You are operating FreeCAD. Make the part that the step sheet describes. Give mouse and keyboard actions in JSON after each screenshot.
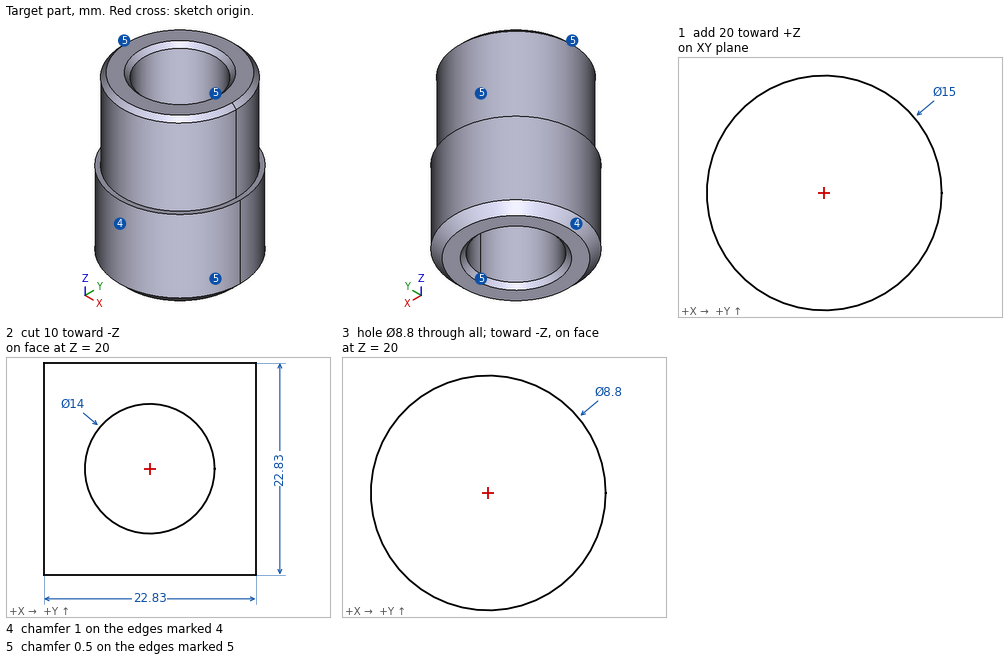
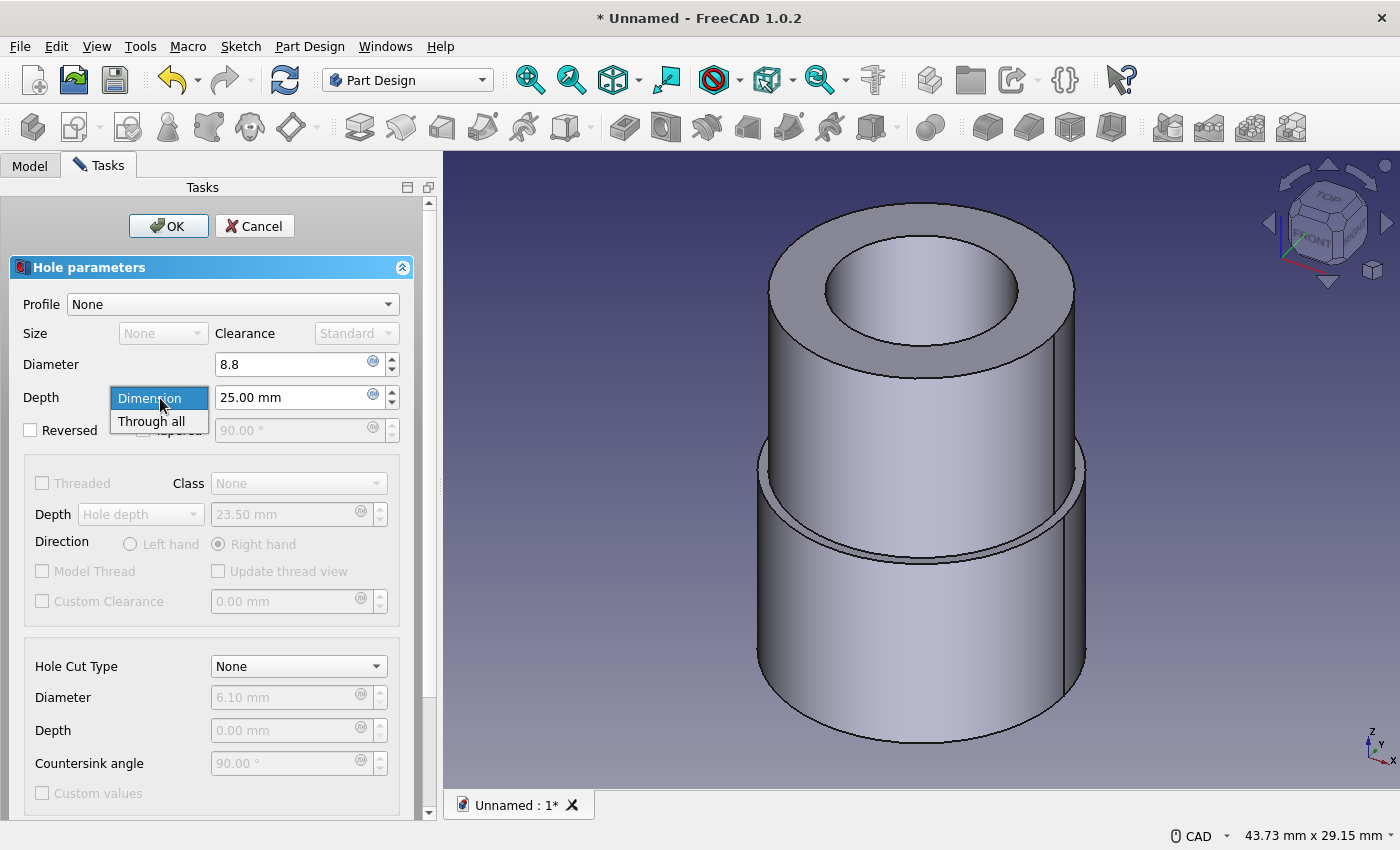
{"action": "left_click", "coordinate": [158, 422]}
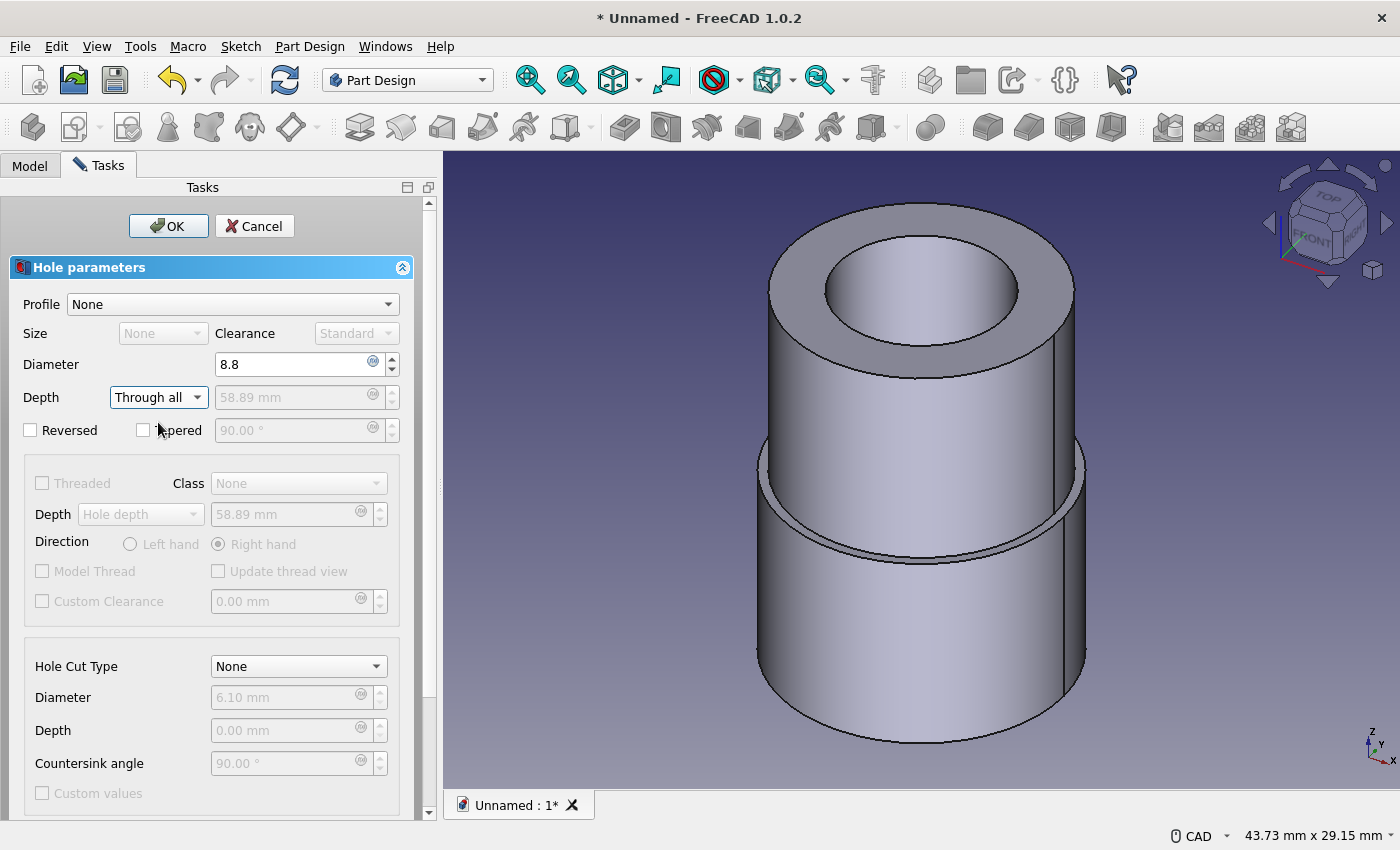
{"action": "left_click", "coordinate": [169, 226]}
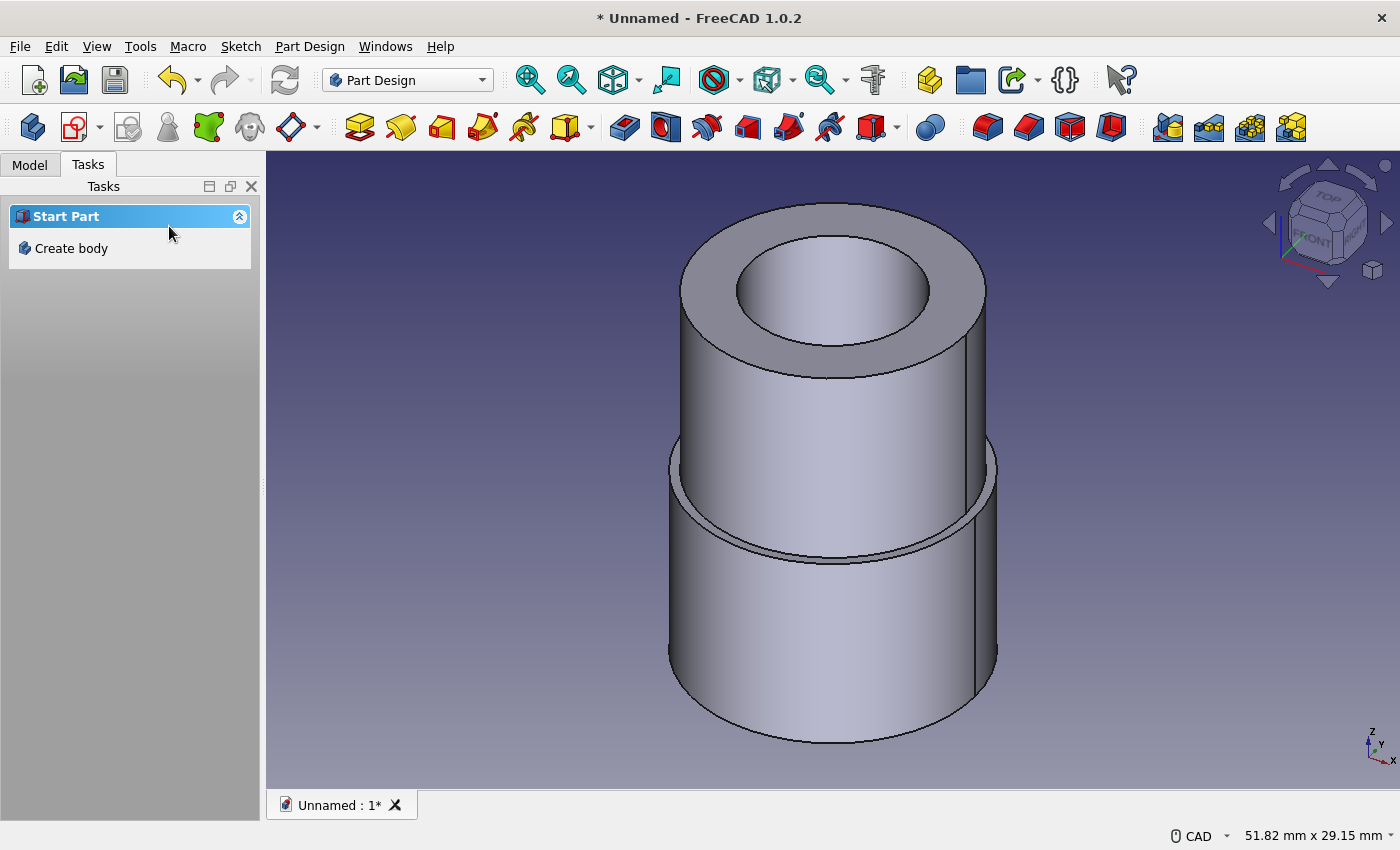
{"action": "key", "text": "0"}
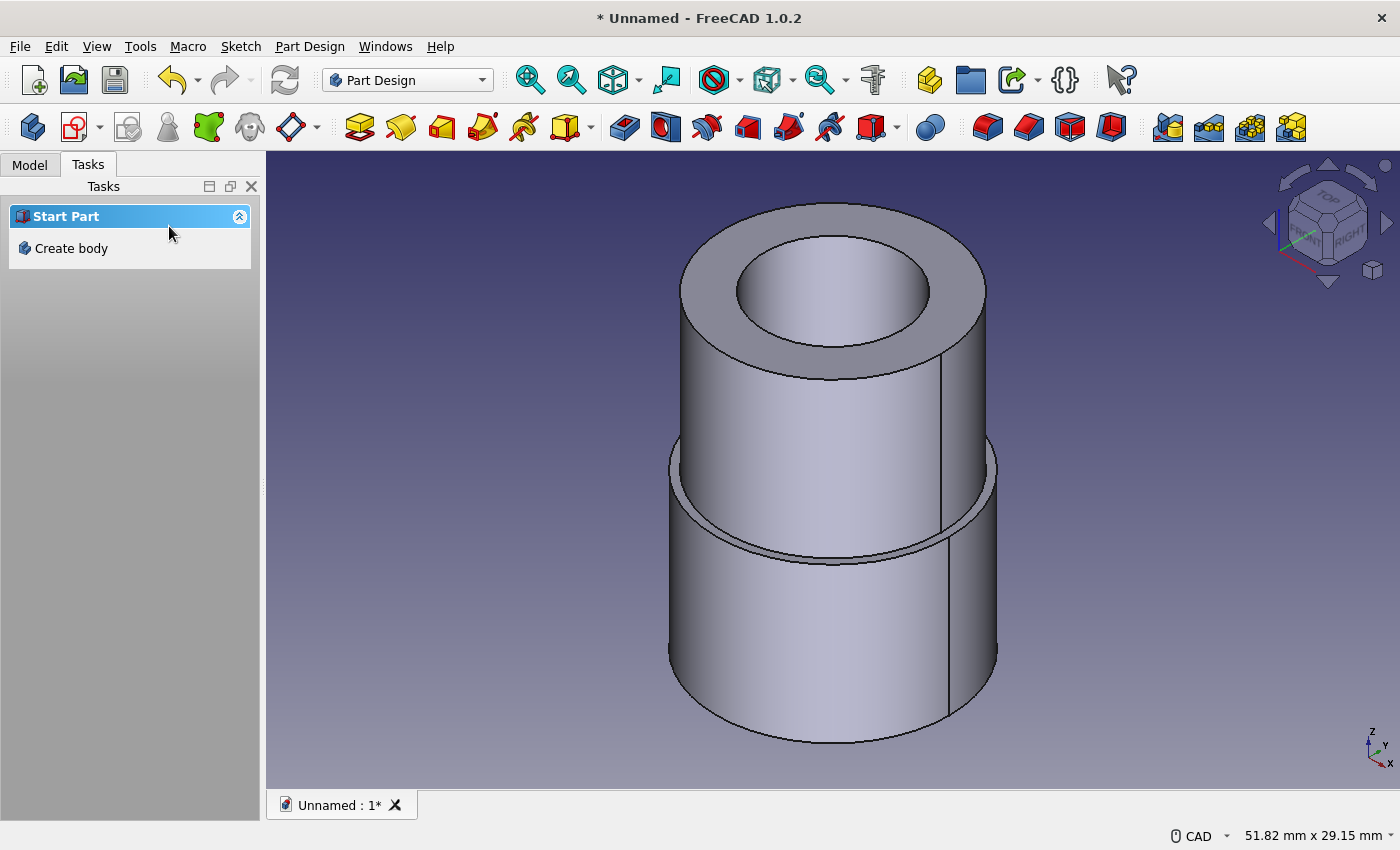
{"action": "key", "text": "2"}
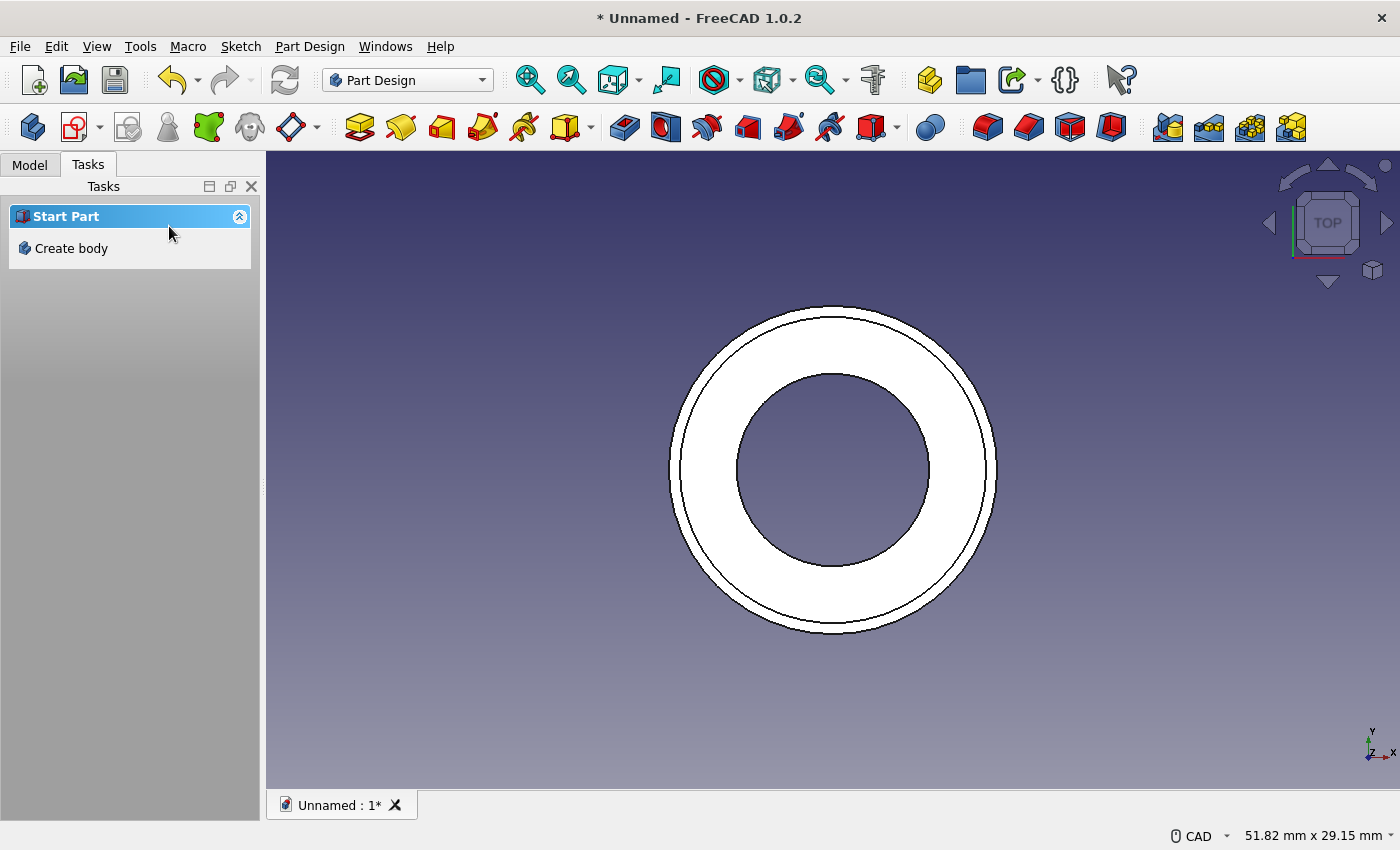
{"action": "key", "text": "1"}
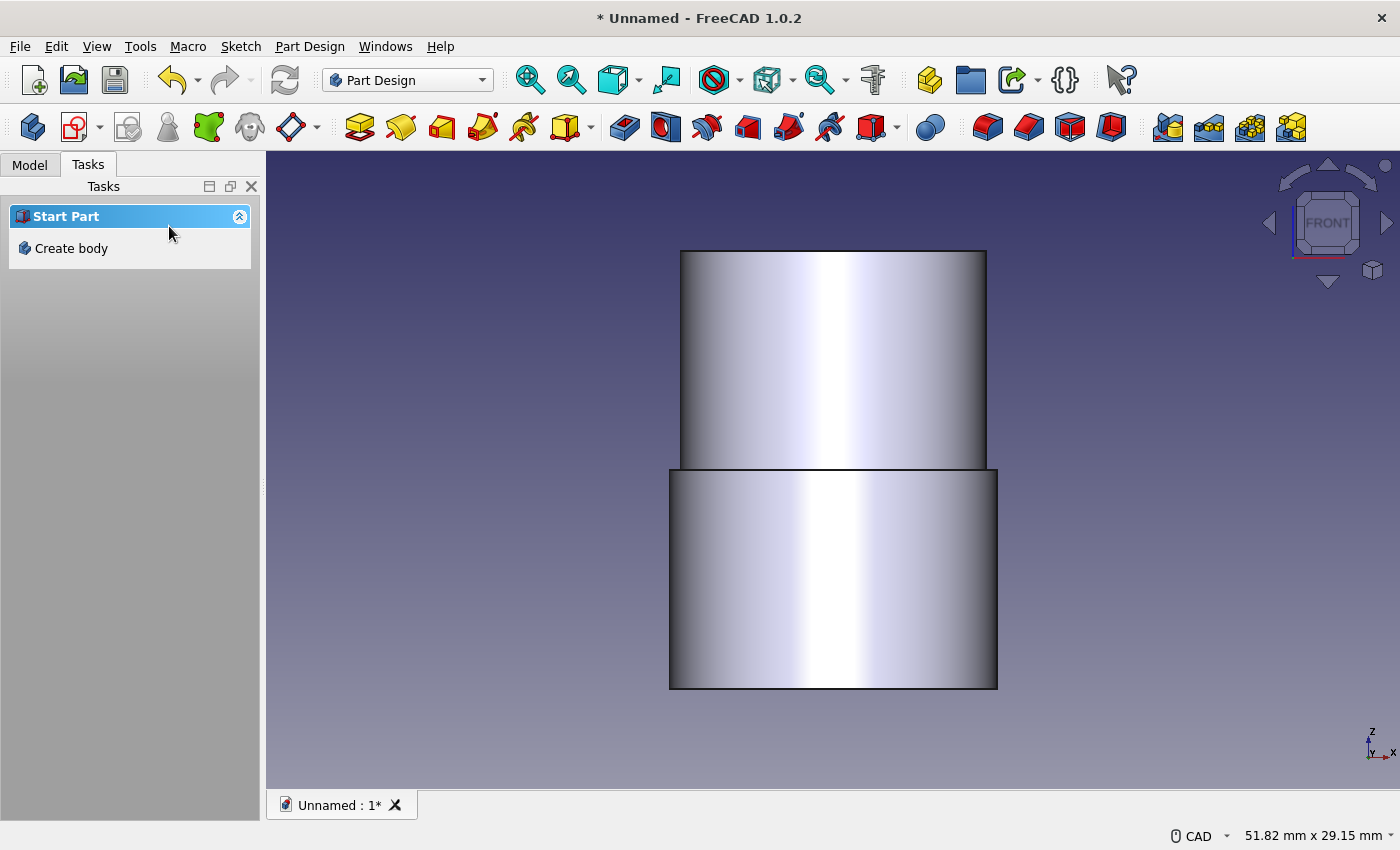
{"action": "left_click", "coordinate": [700, 688]}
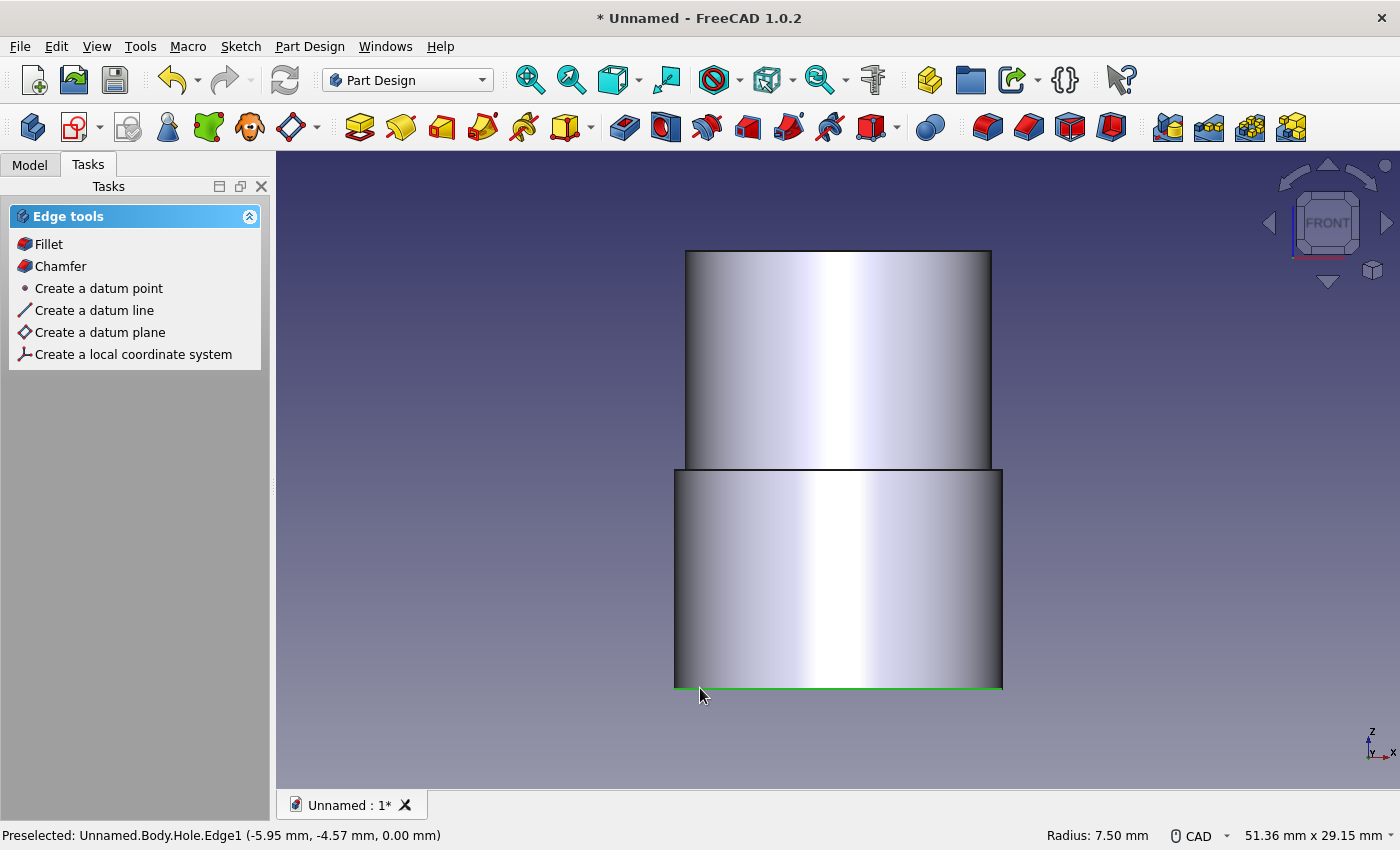
{"action": "left_click", "coordinate": [1029, 128]}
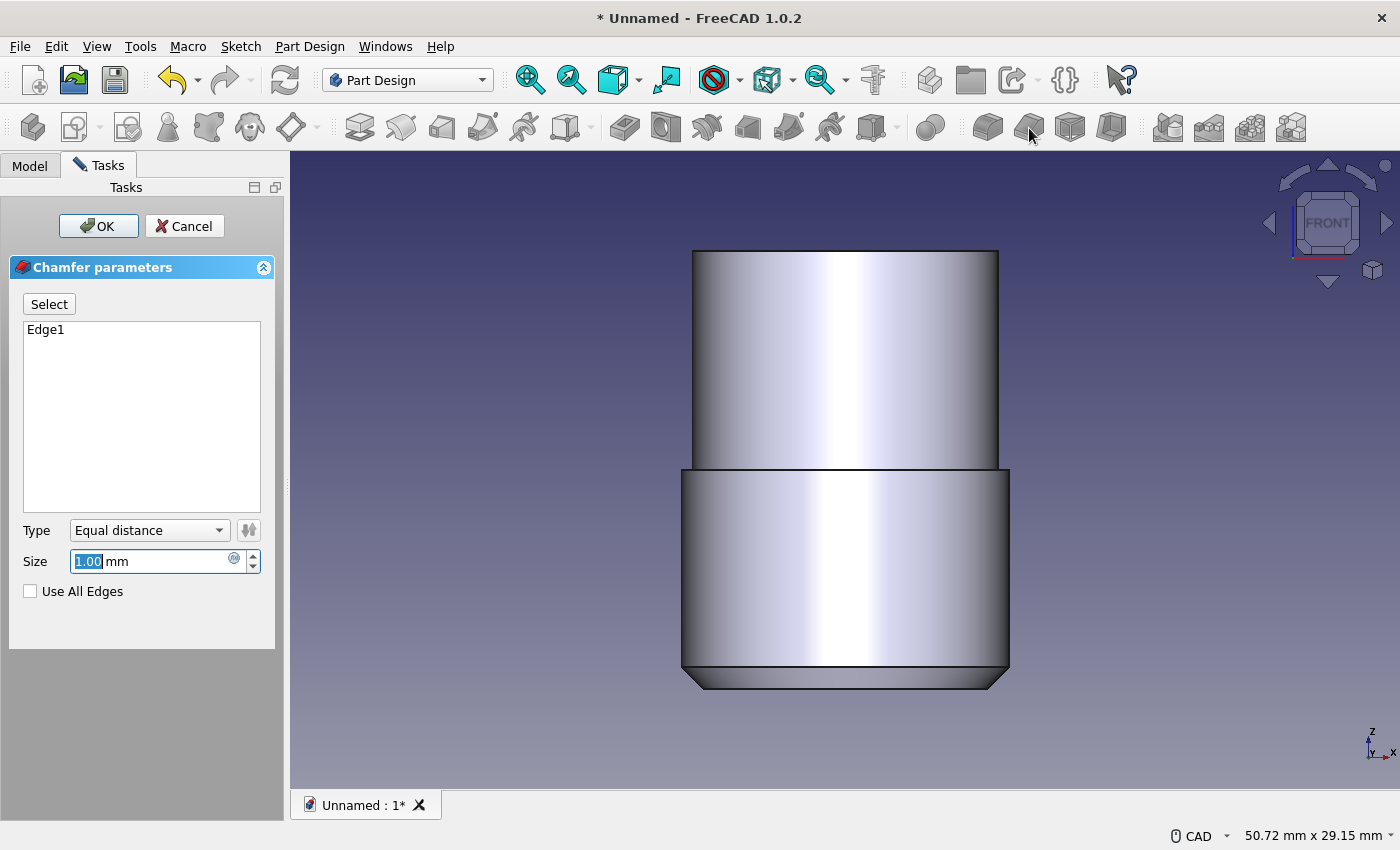
{"action": "type", "text": "1"}
{"action": "key", "text": "Tab"}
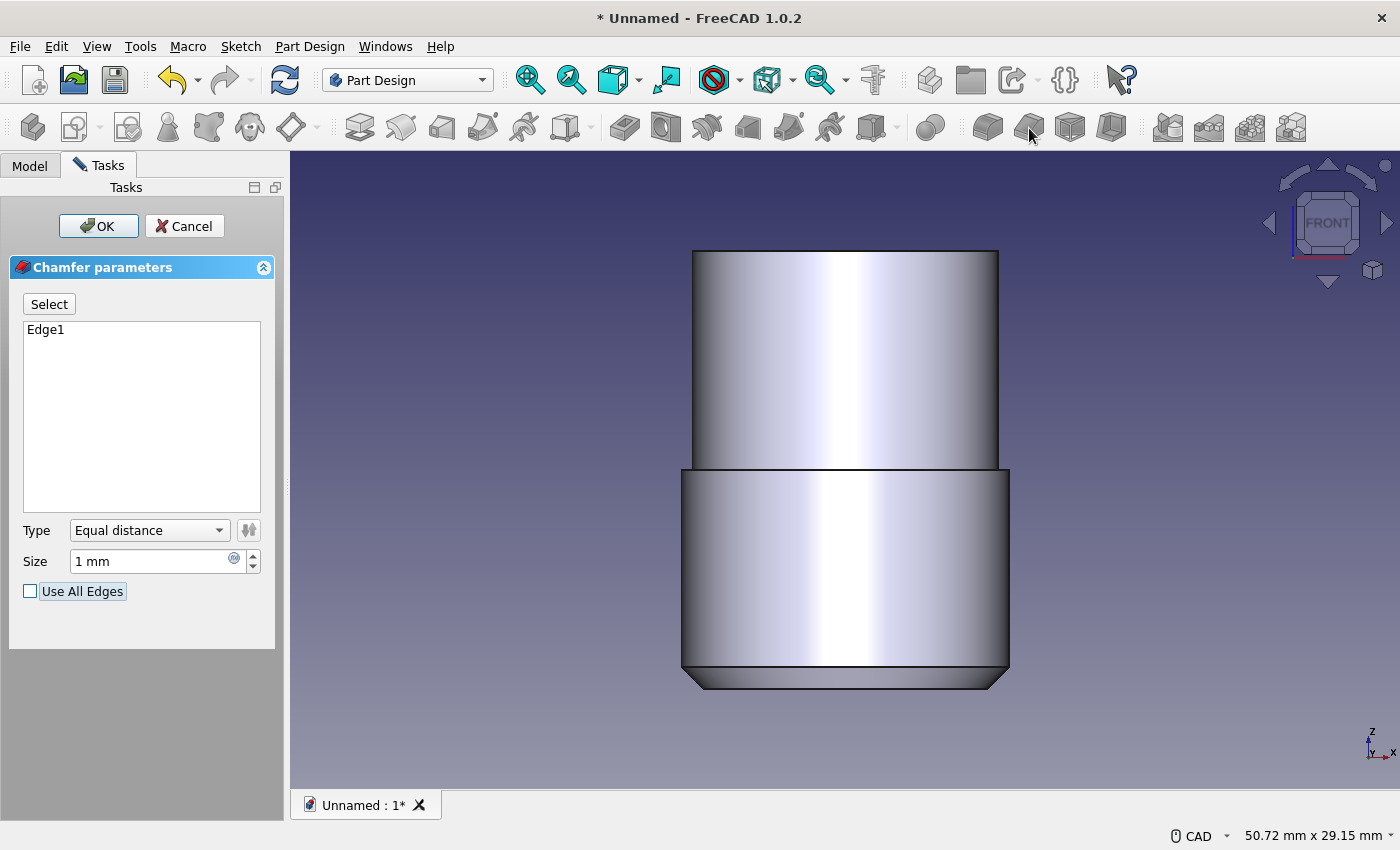
{"action": "left_click", "coordinate": [99, 226]}